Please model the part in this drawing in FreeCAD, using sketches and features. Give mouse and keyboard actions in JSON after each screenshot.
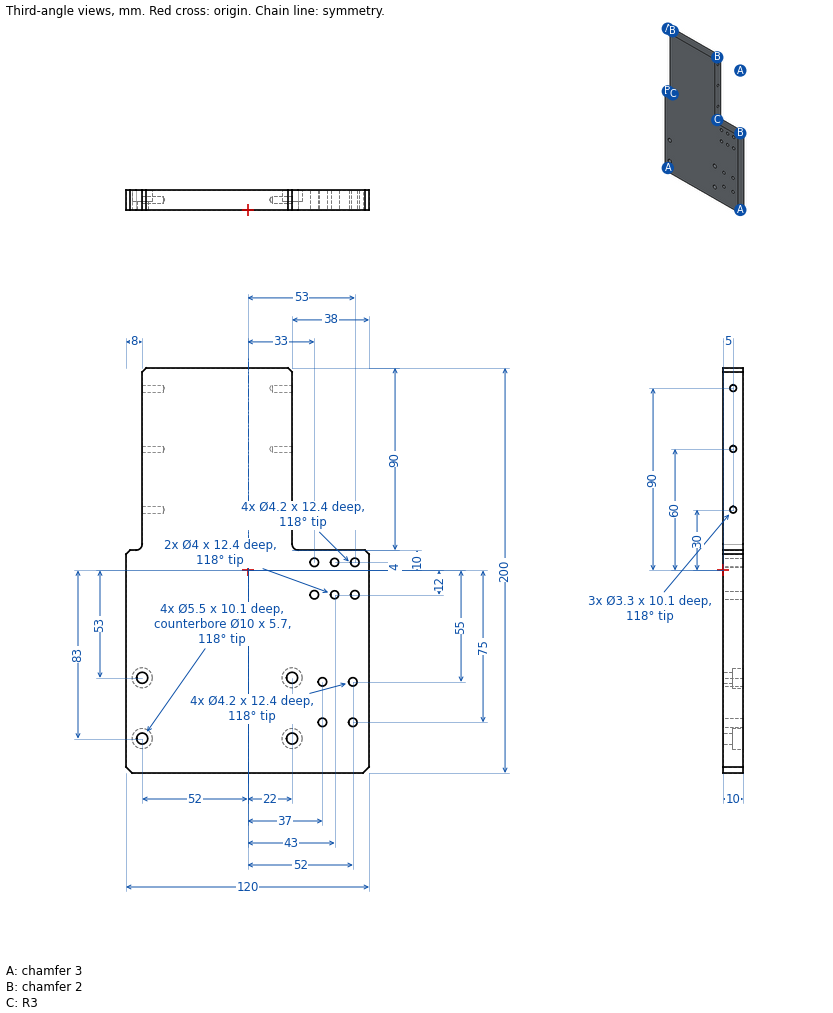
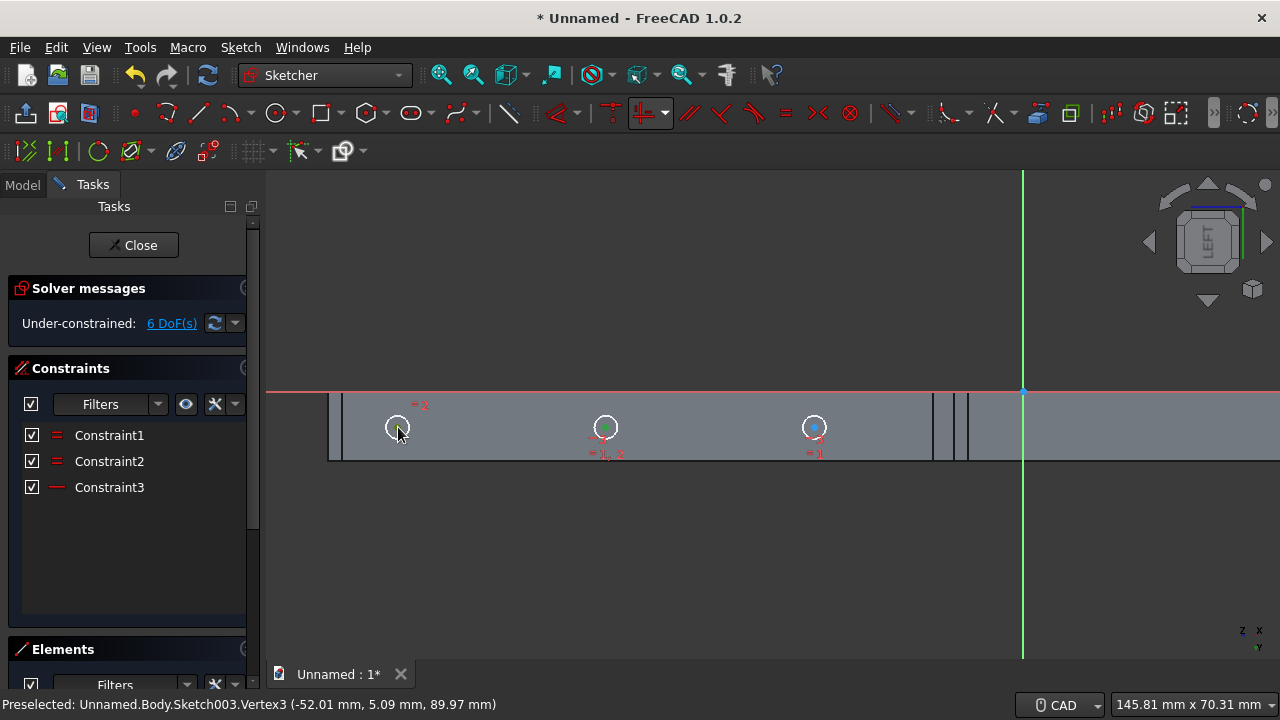
{"action": "left_click", "coordinate": [668, 114]}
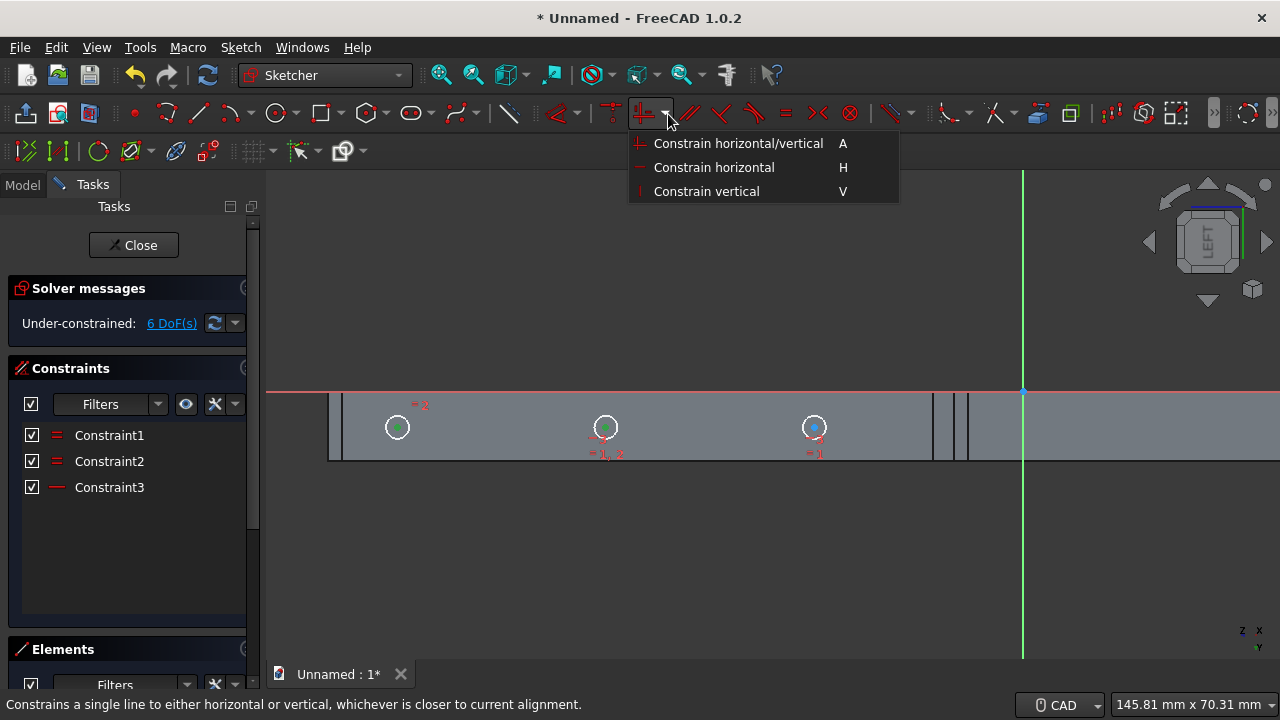
{"action": "left_click", "coordinate": [764, 167]}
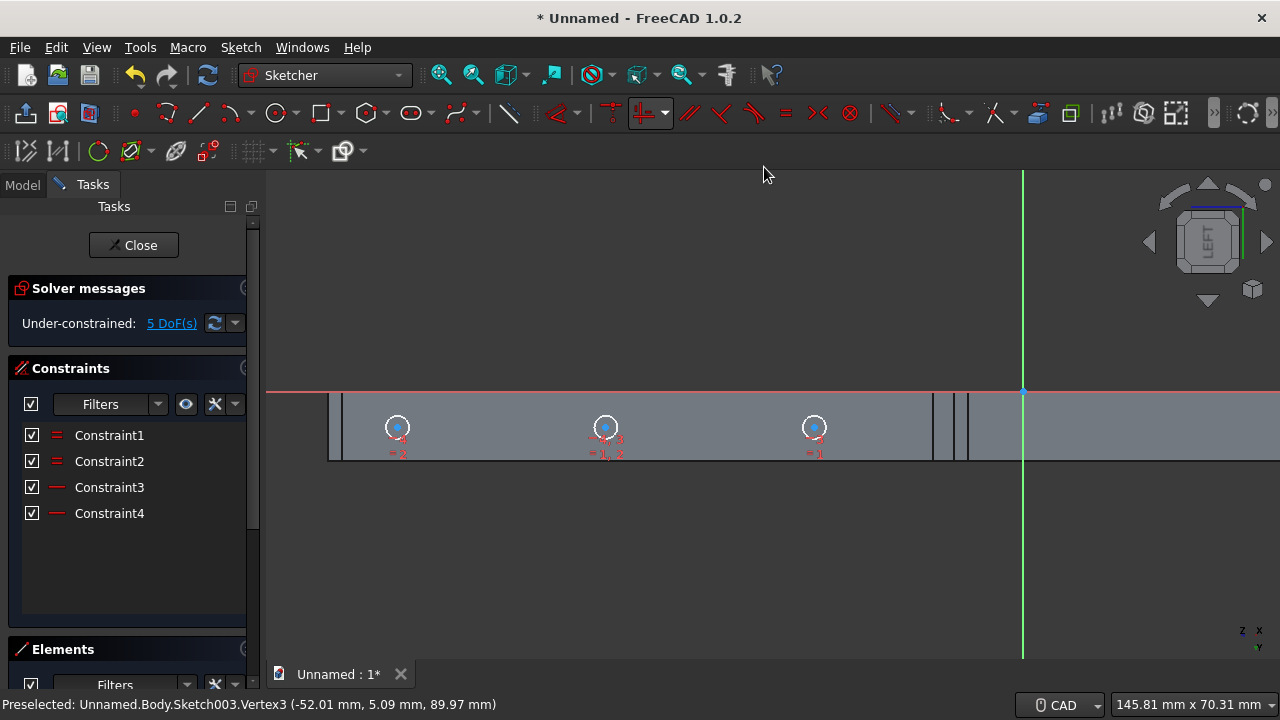
{"action": "key", "text": "d"}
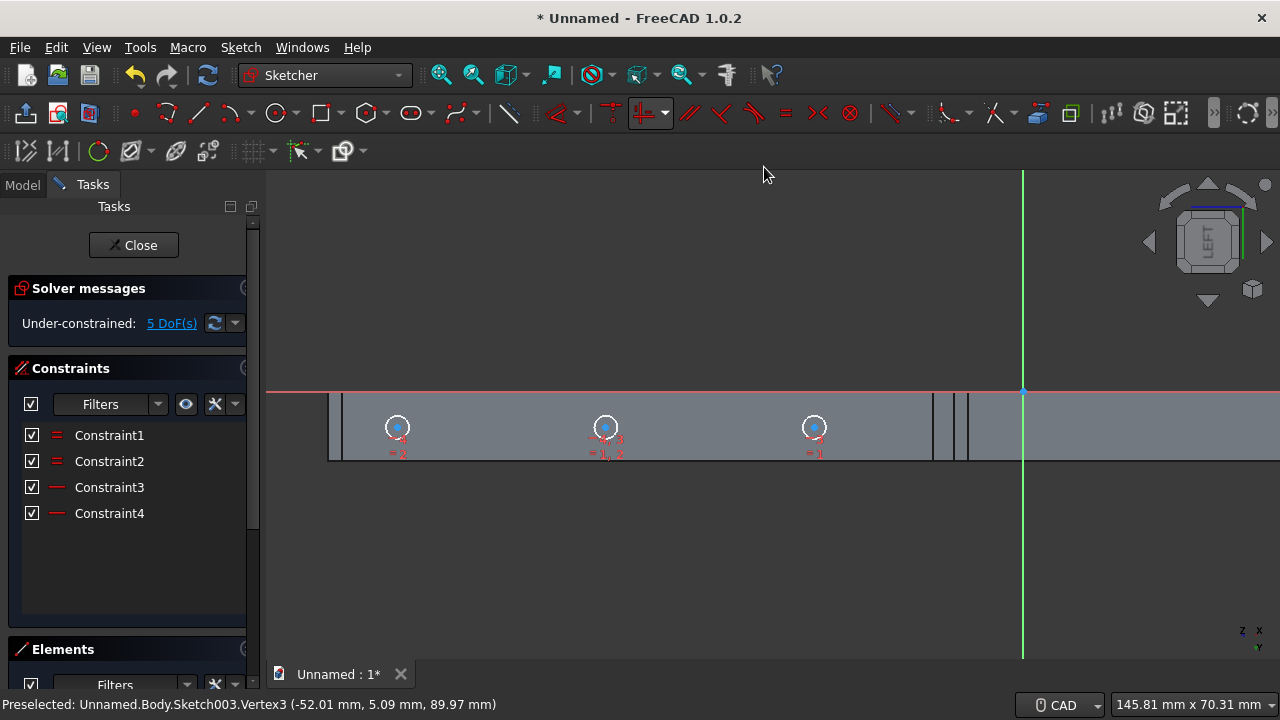
{"action": "scroll", "coordinate": [822, 419], "scroll_direction": "up", "scroll_amount": 3}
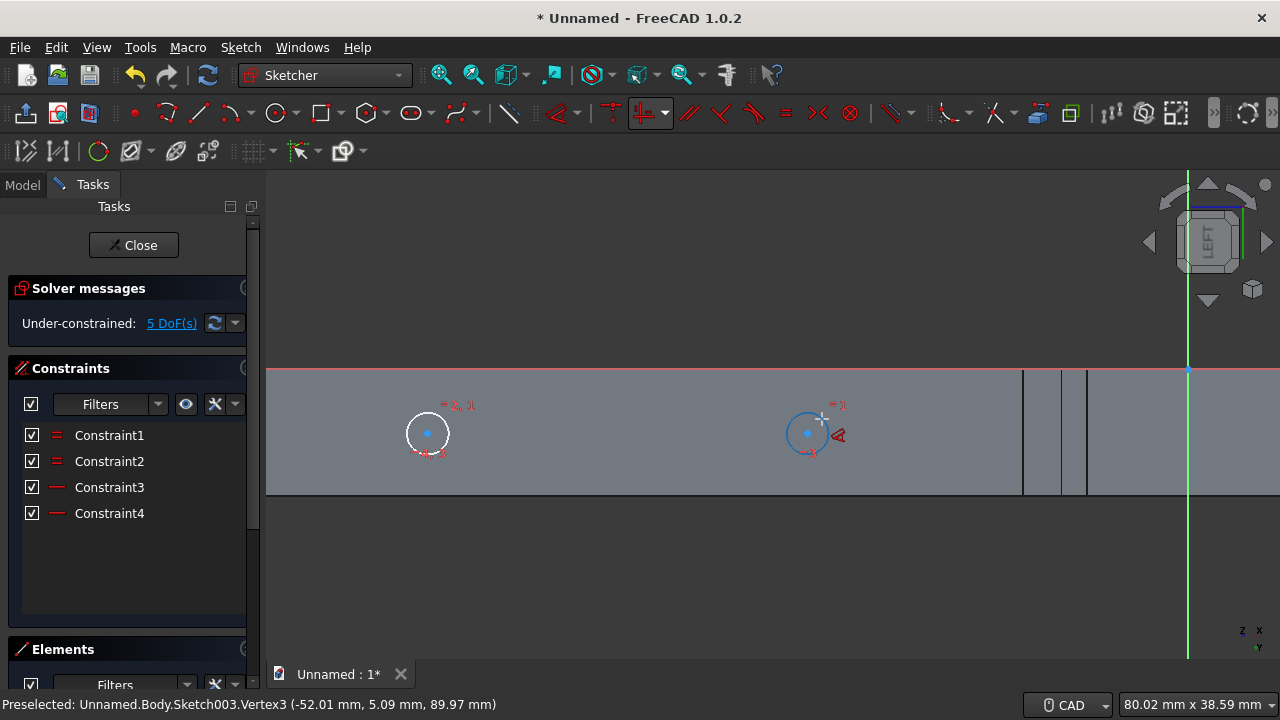
{"action": "left_click", "coordinate": [822, 419]}
{"action": "left_click", "coordinate": [844, 396]}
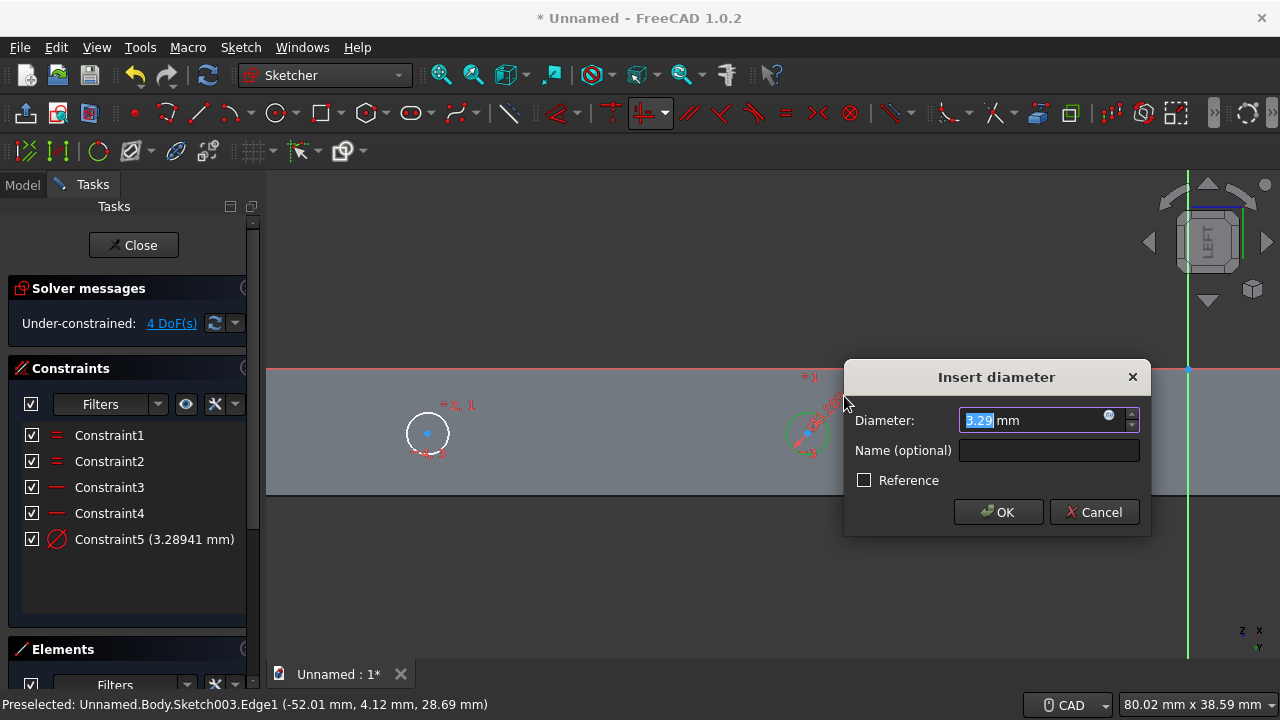
{"action": "type", "text": "3.3"}
{"action": "key", "text": "Return"}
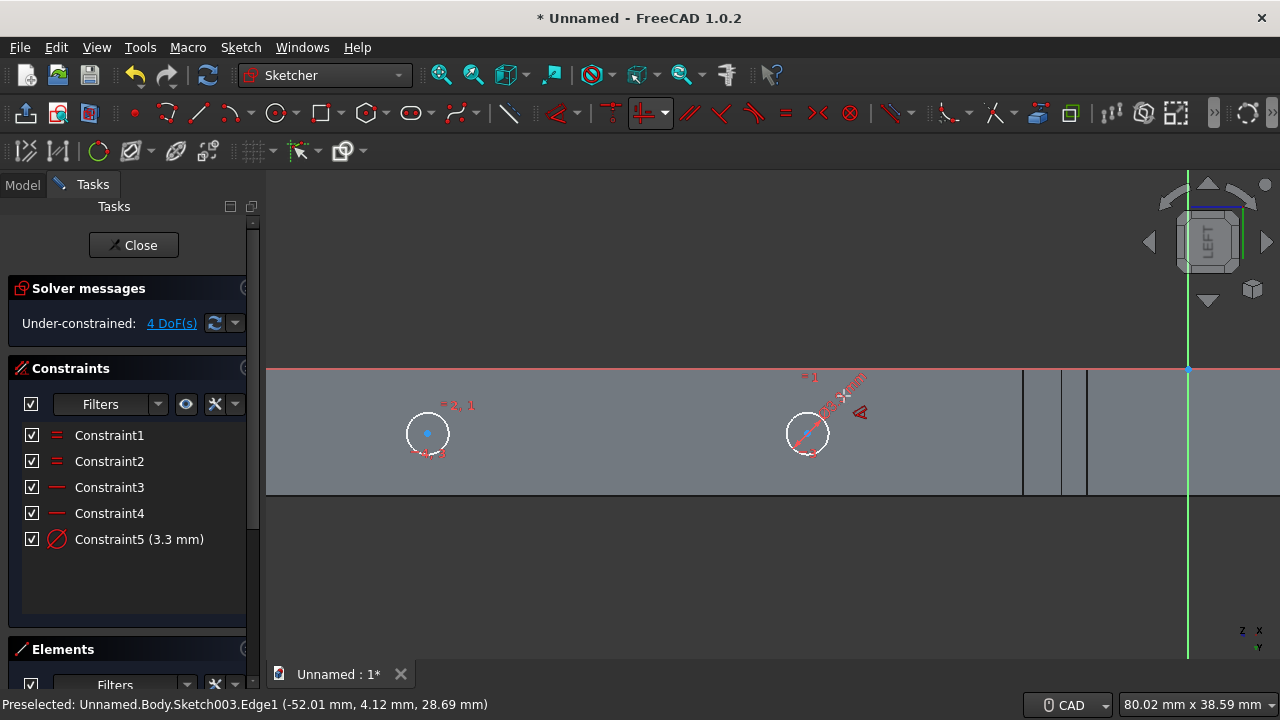
{"action": "left_click", "coordinate": [808, 434]}
{"action": "left_click", "coordinate": [774, 401]}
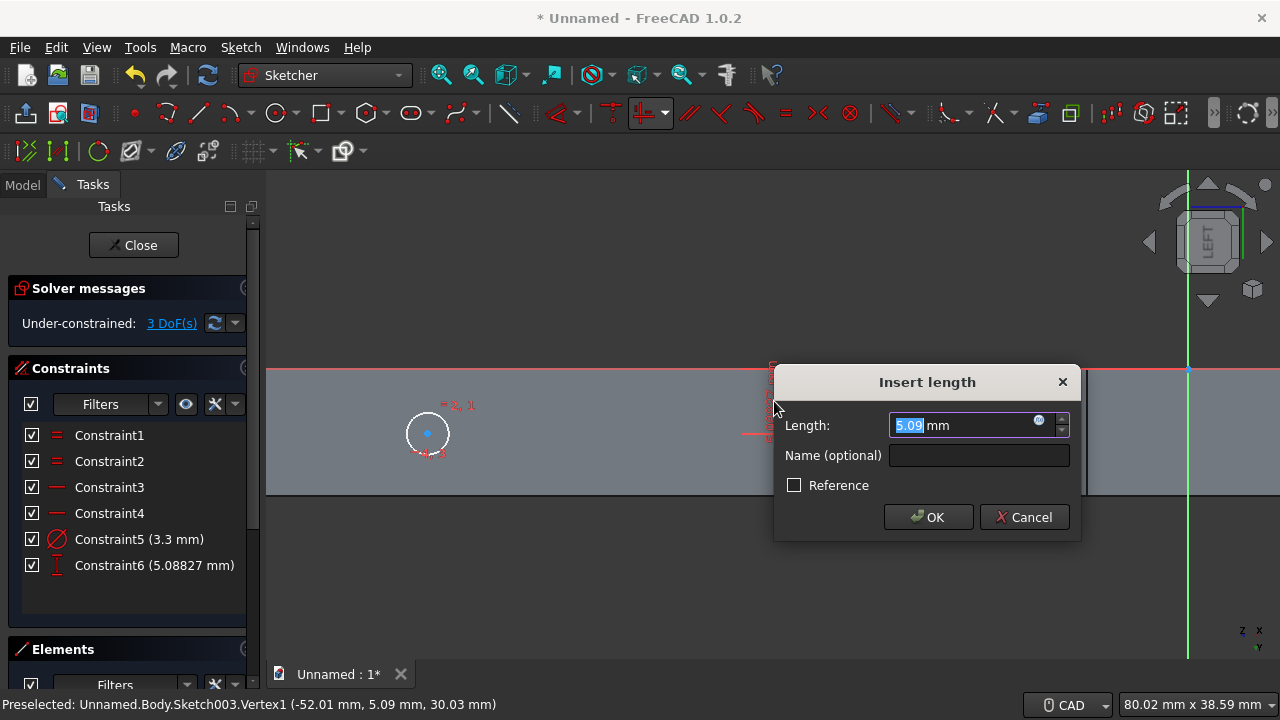
{"action": "type", "text": "5"}
{"action": "key", "text": "Return"}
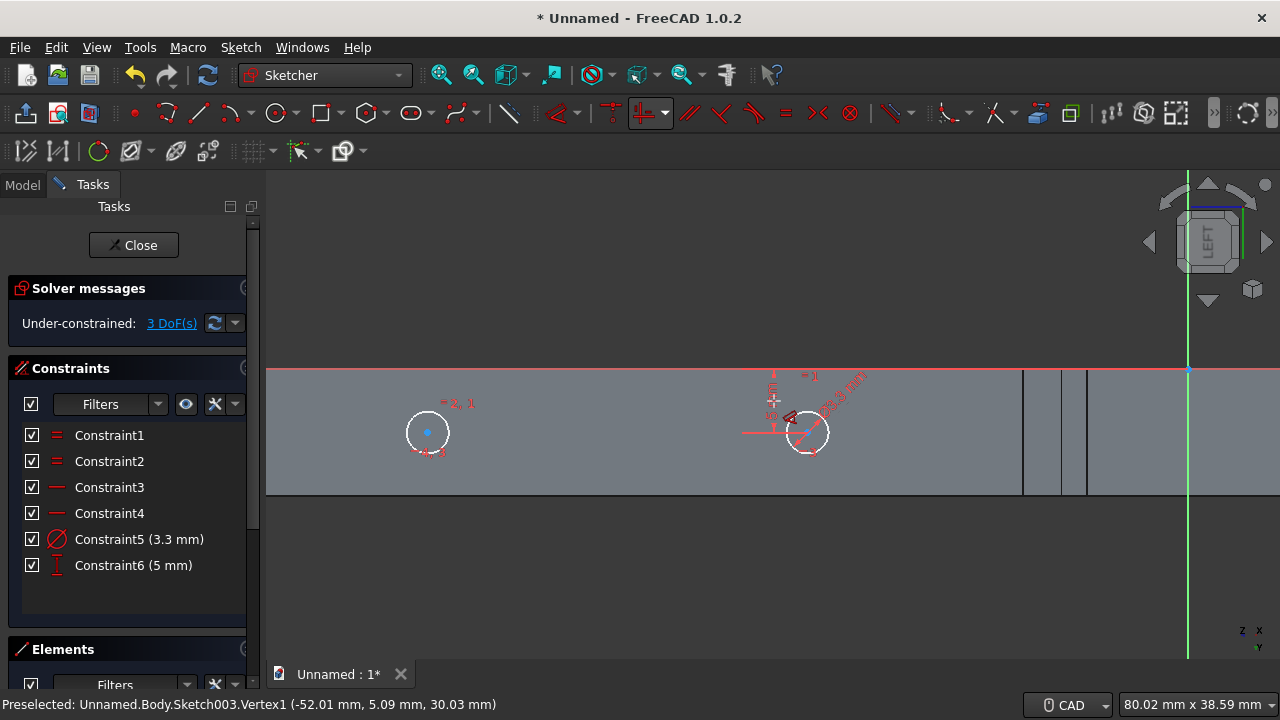
{"action": "left_click", "coordinate": [808, 433]}
{"action": "left_click", "coordinate": [961, 335]}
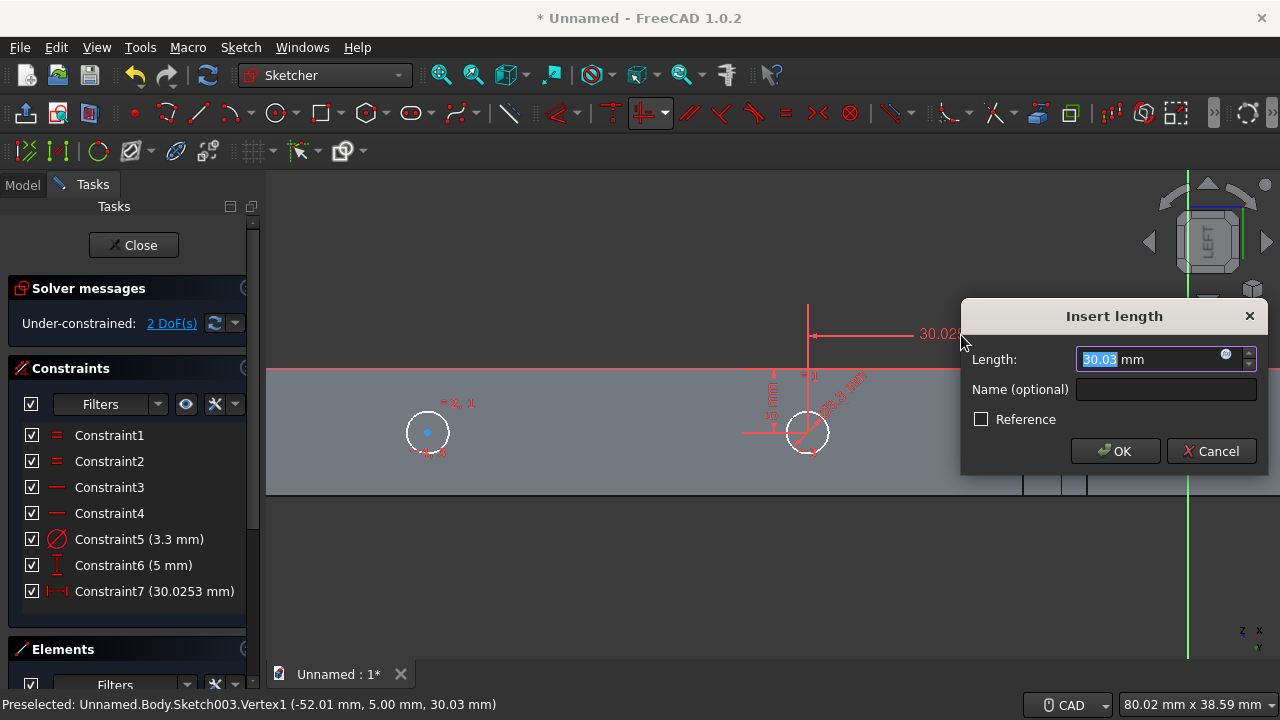
{"action": "type", "text": "30"}
{"action": "key", "text": "Return"}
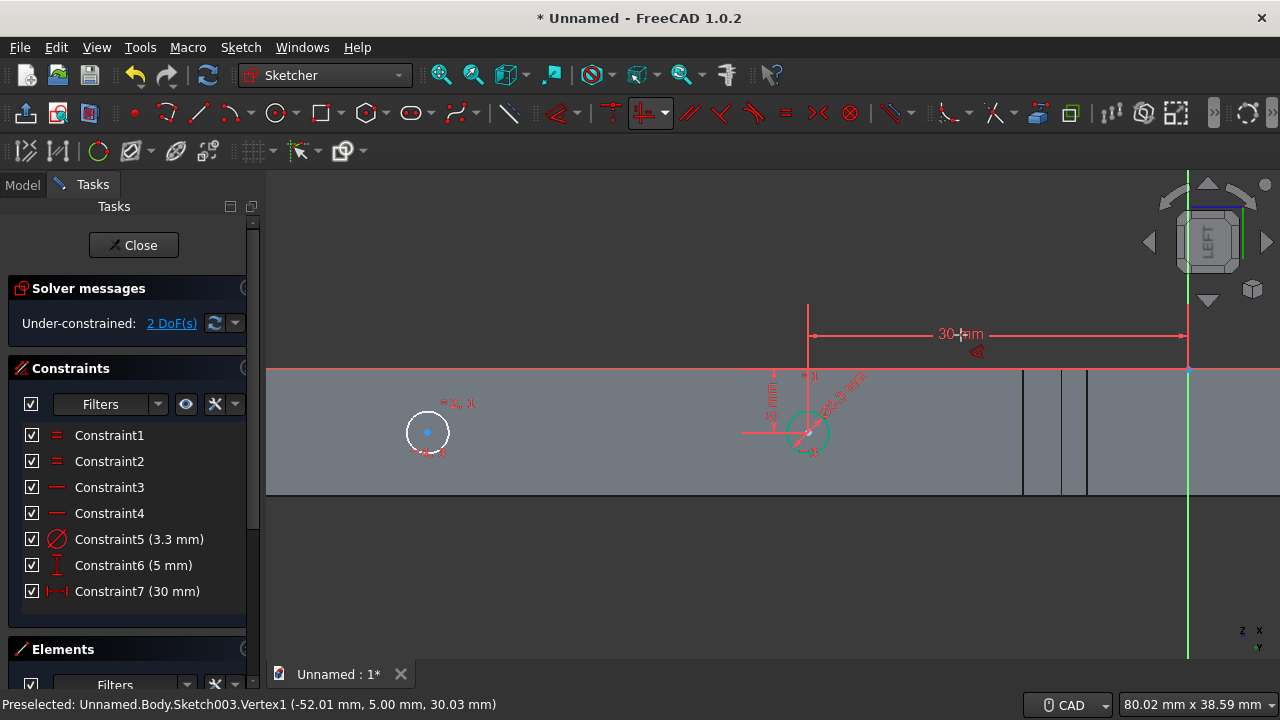
{"action": "left_click", "coordinate": [428, 433]}
{"action": "left_click", "coordinate": [771, 335]}